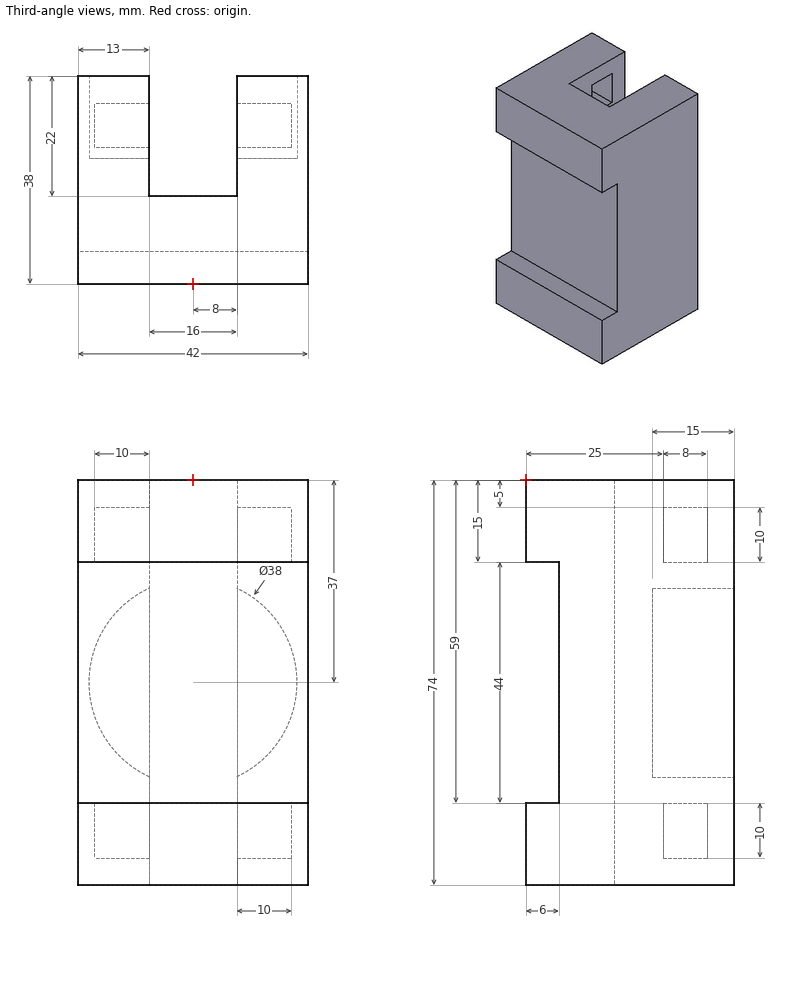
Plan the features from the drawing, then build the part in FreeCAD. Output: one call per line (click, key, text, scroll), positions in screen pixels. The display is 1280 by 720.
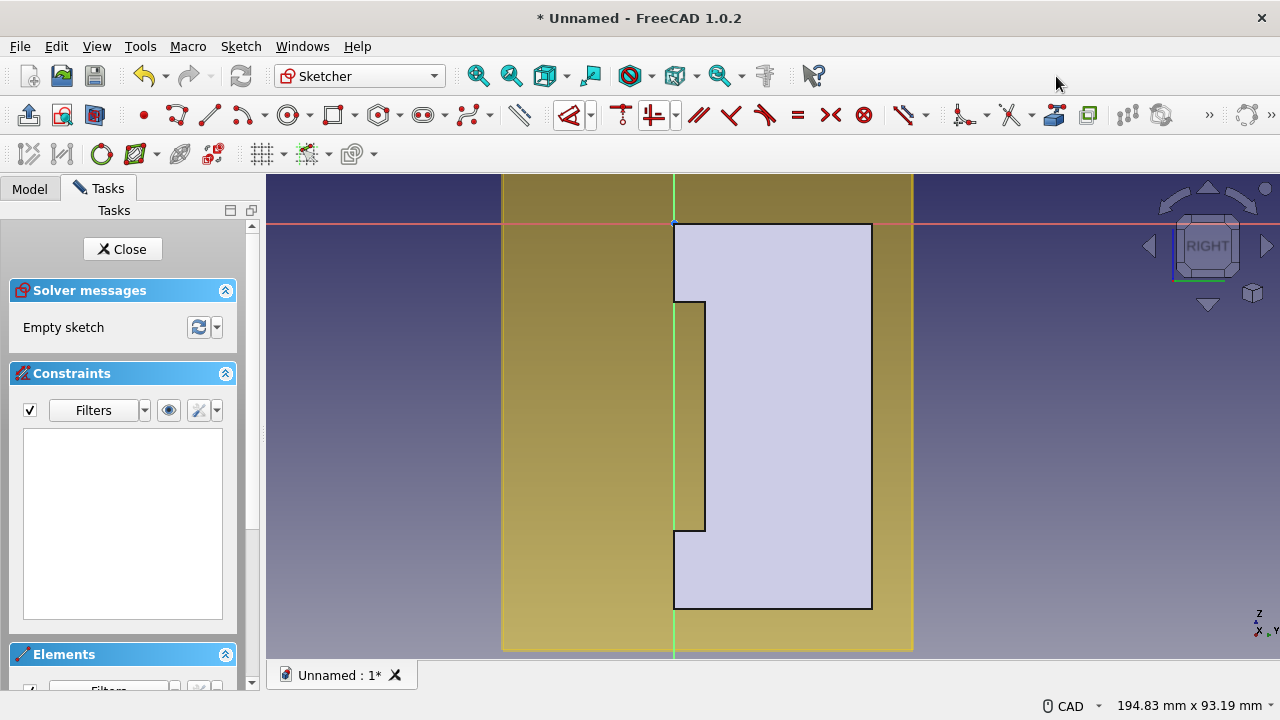
key(q)
key(s)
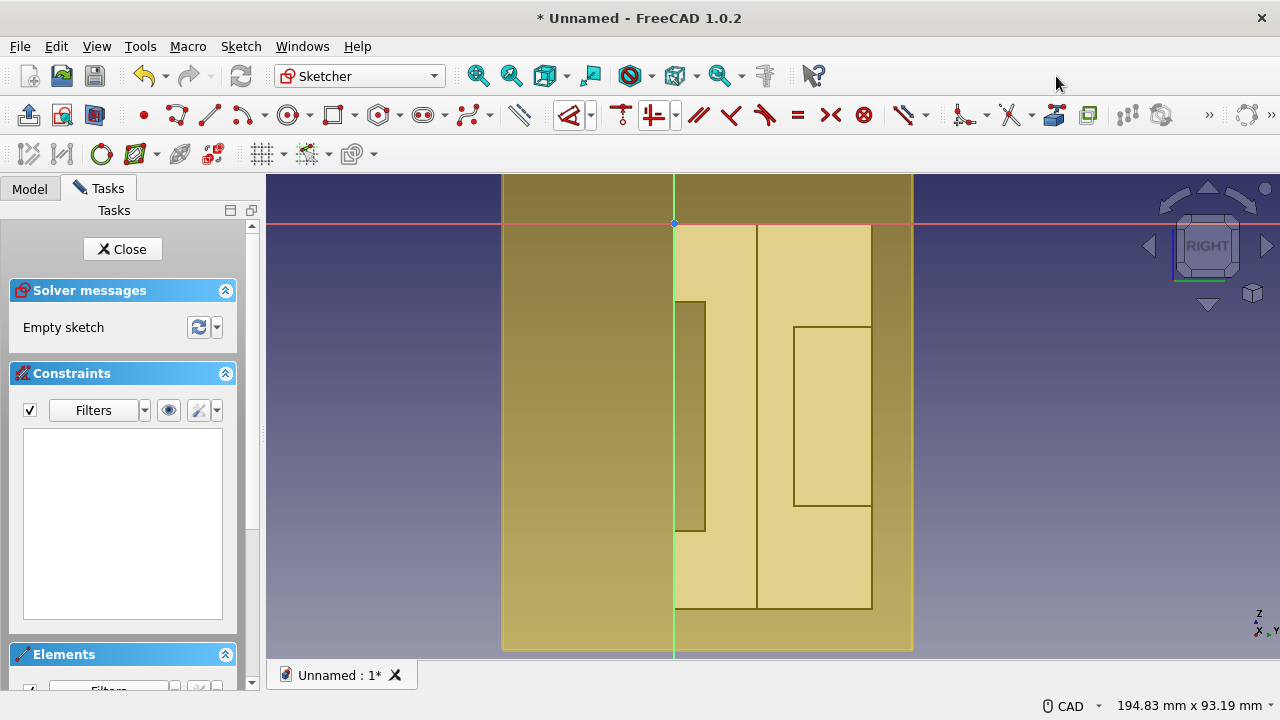
scroll(454, 475, down, 1)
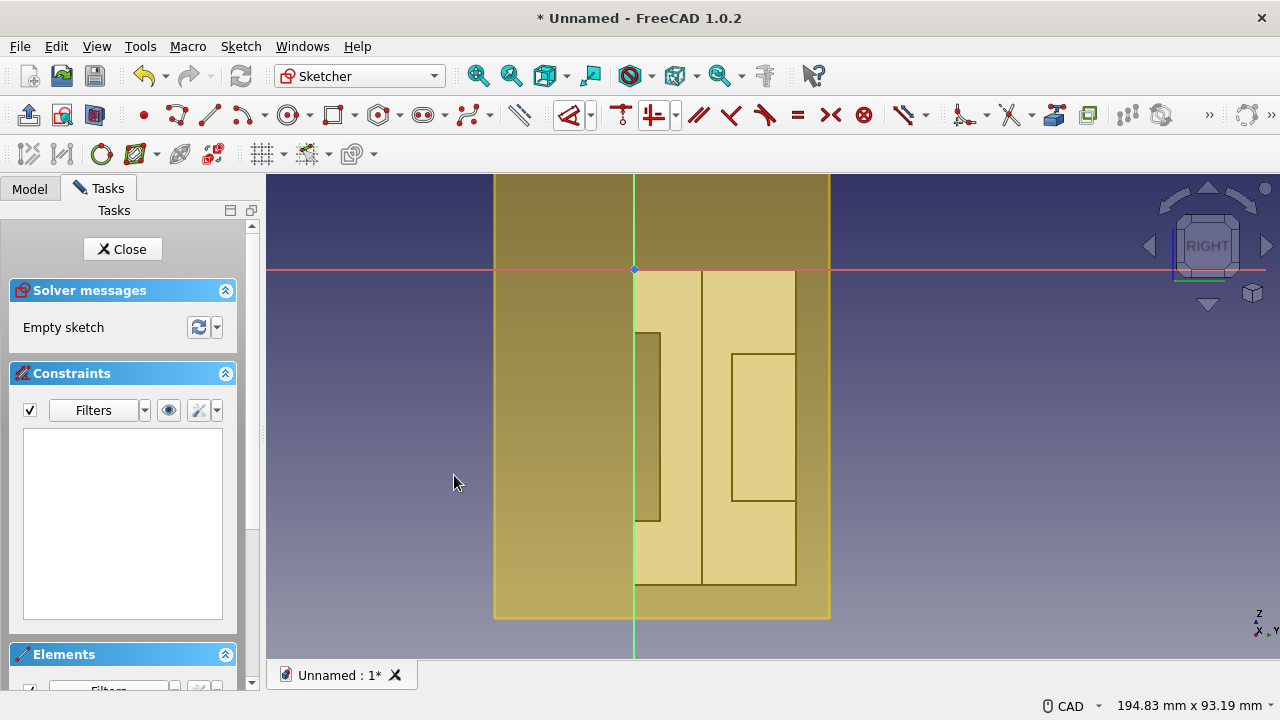
key(g)
key(r)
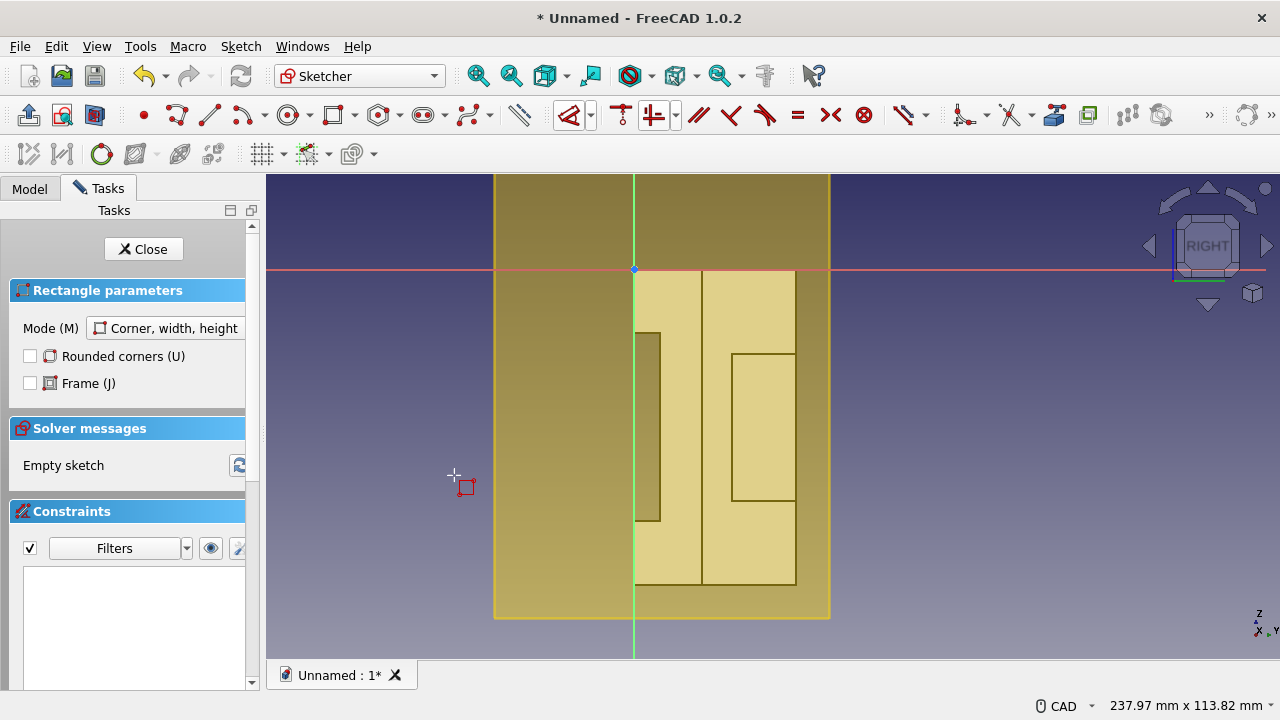
click(741, 291)
move(775, 333)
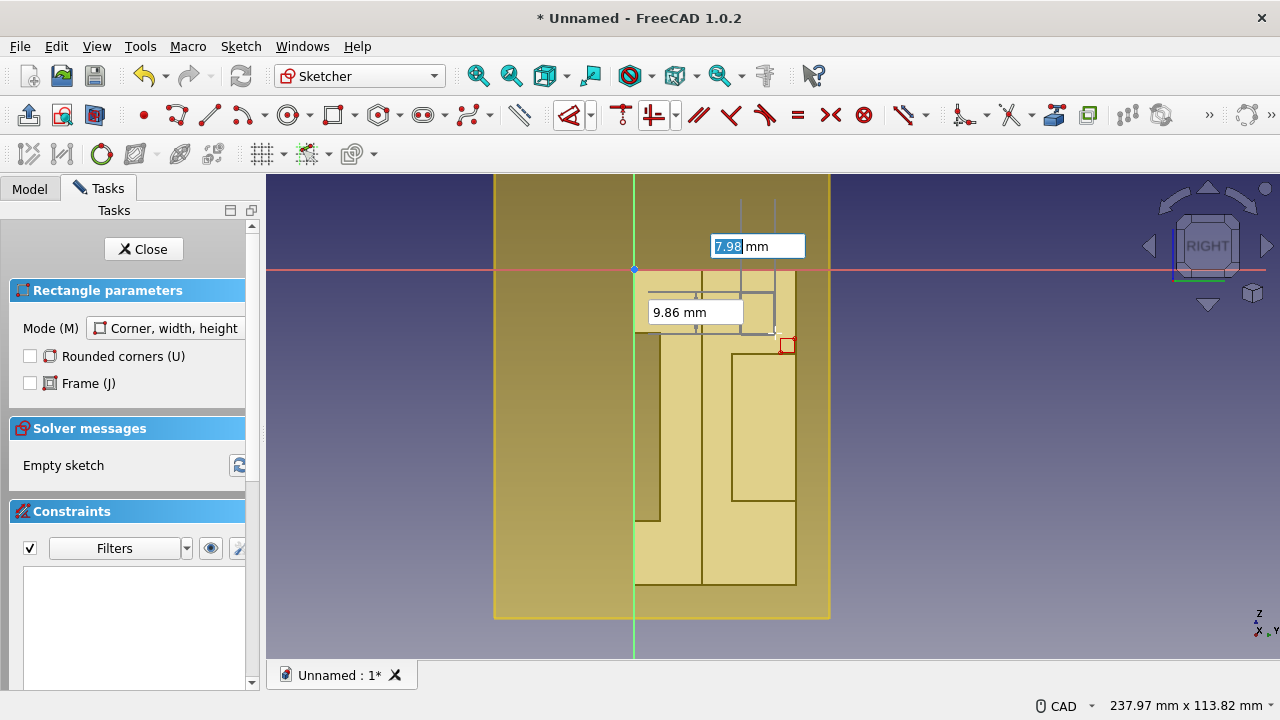
text(8)
key(Tab)
text(10)
key(Return)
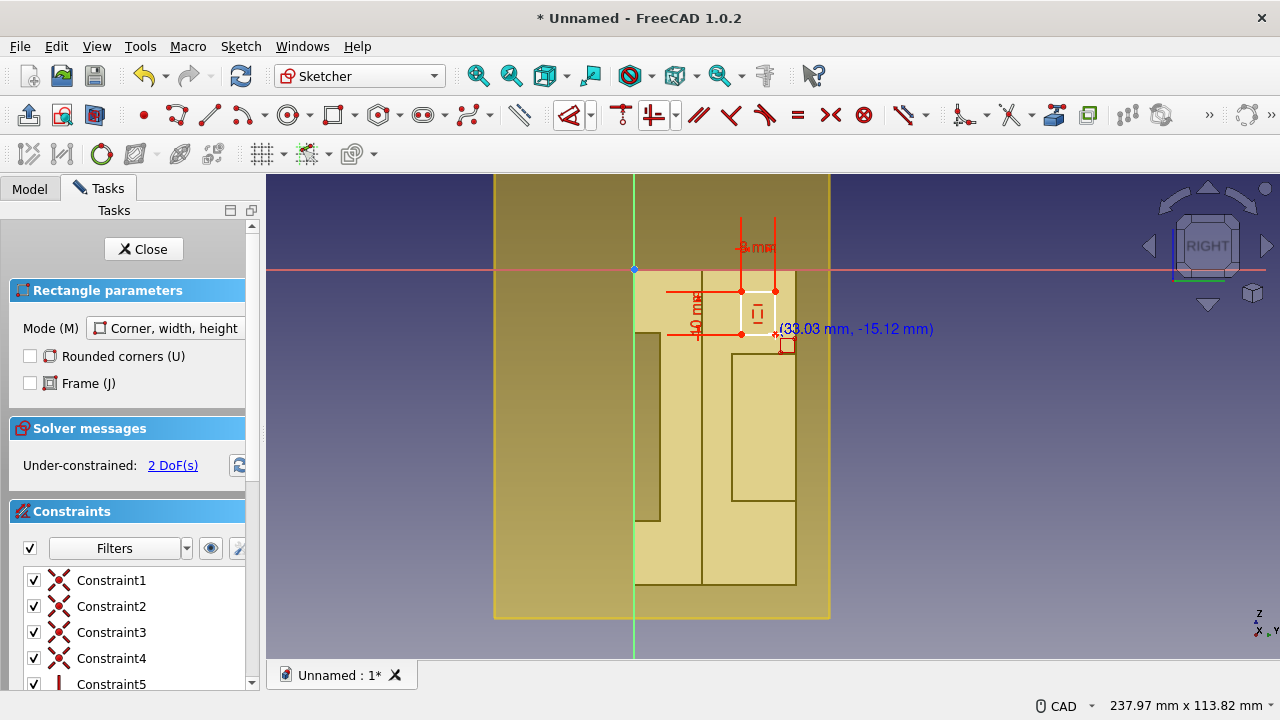
click(741, 521)
move(775, 564)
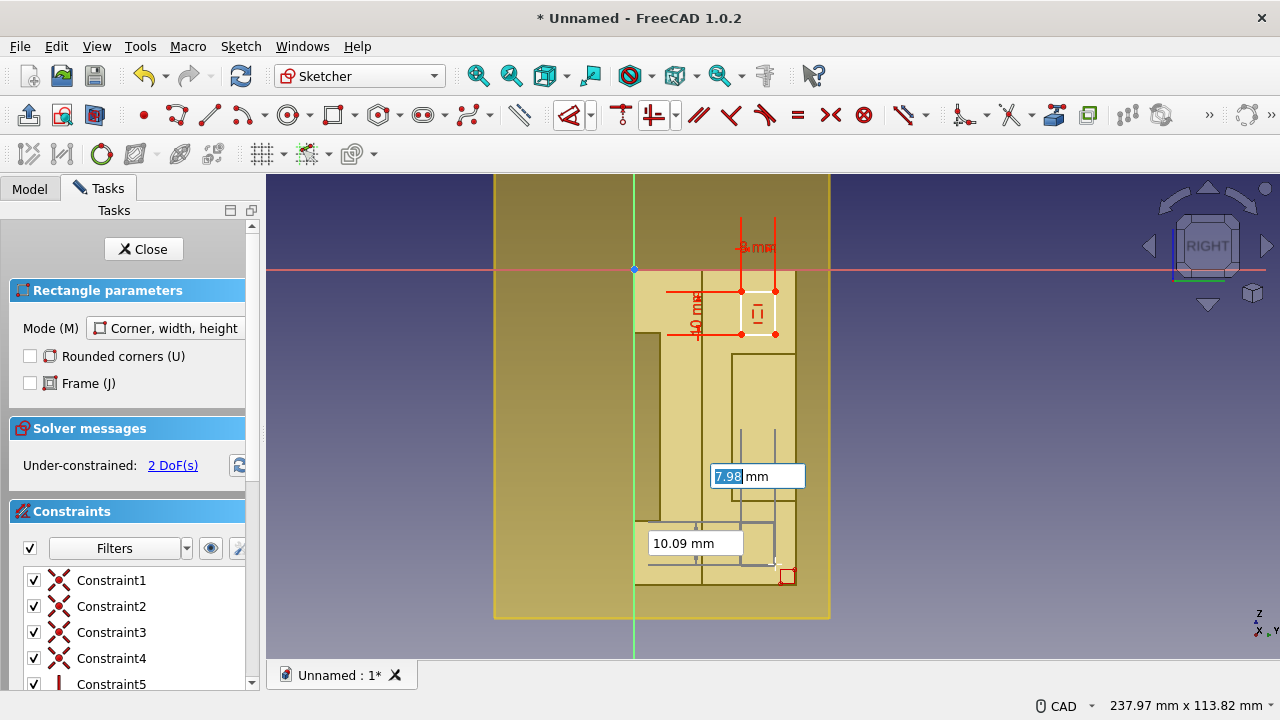
text(8)
key(Tab)
text(10)
key(Return)
key(Escape)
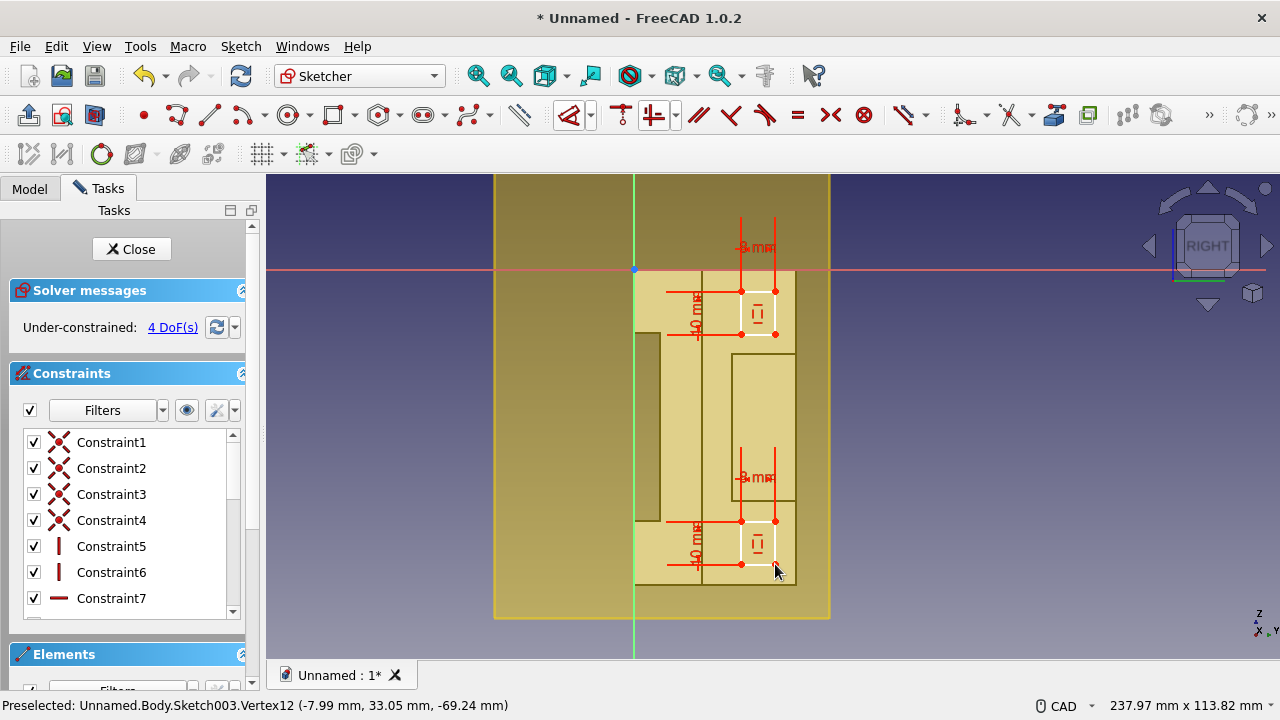
scroll(741, 292, up, 4)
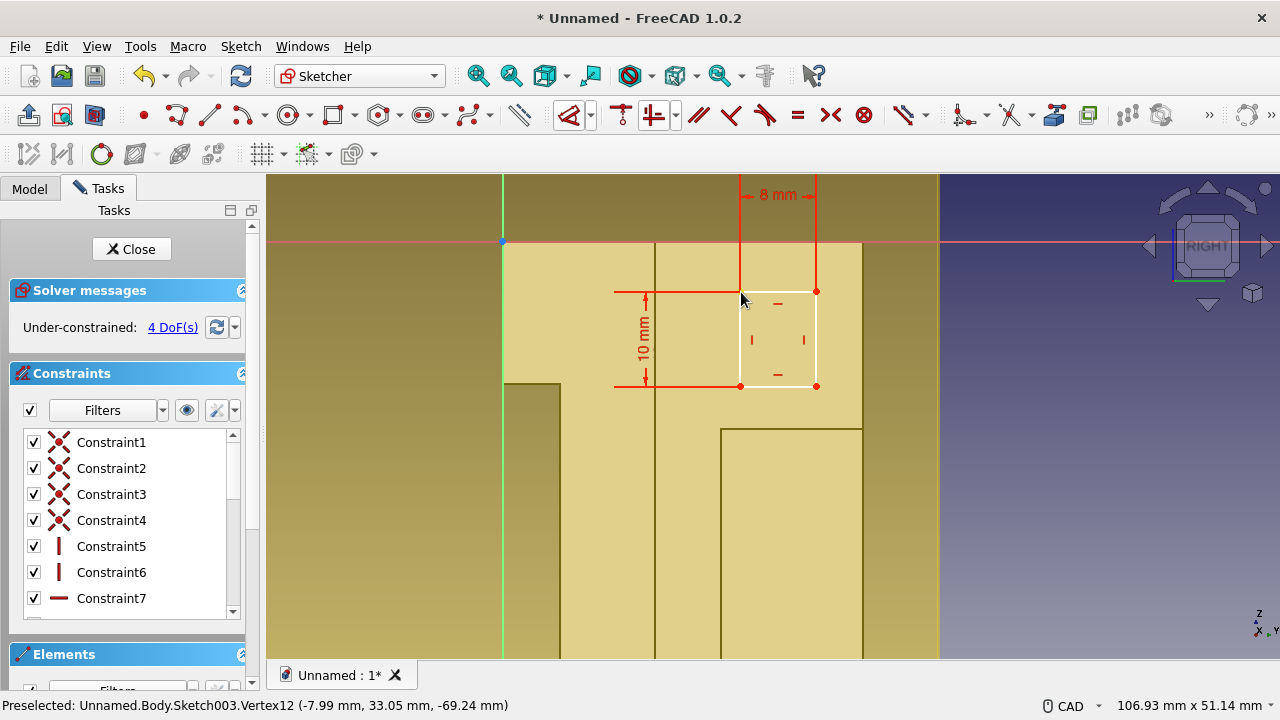
click(740, 292)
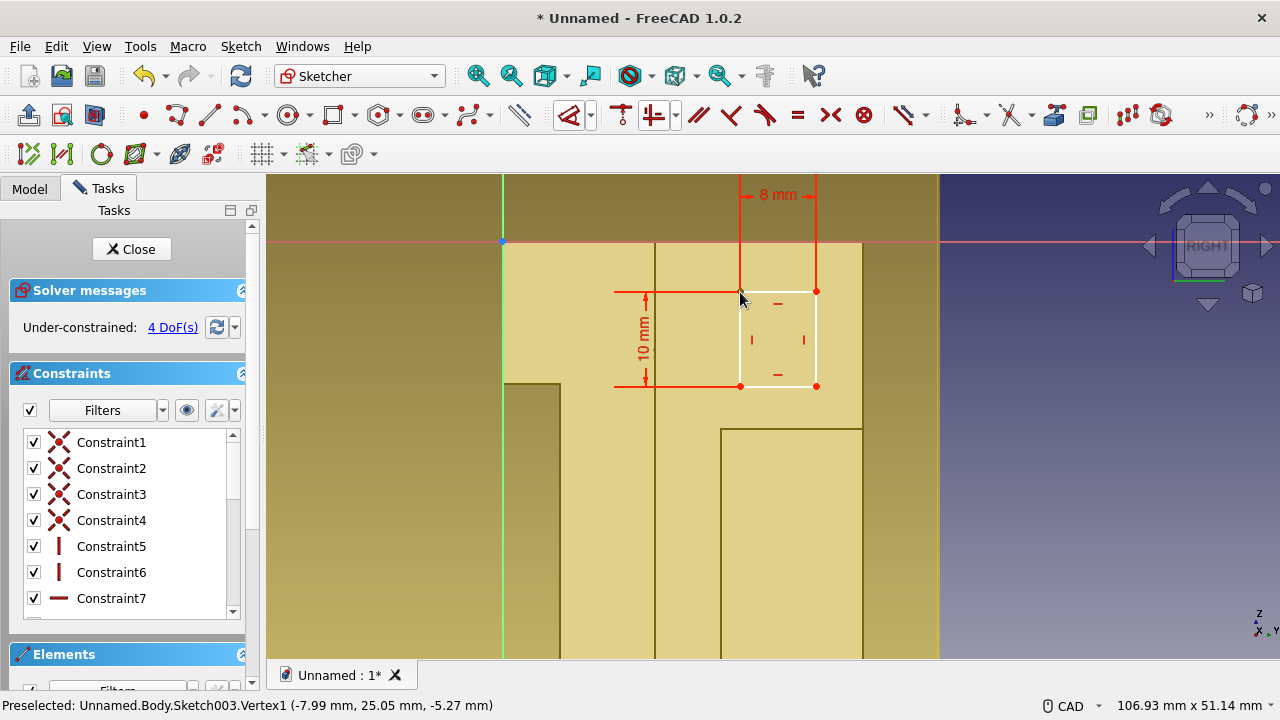
key(i)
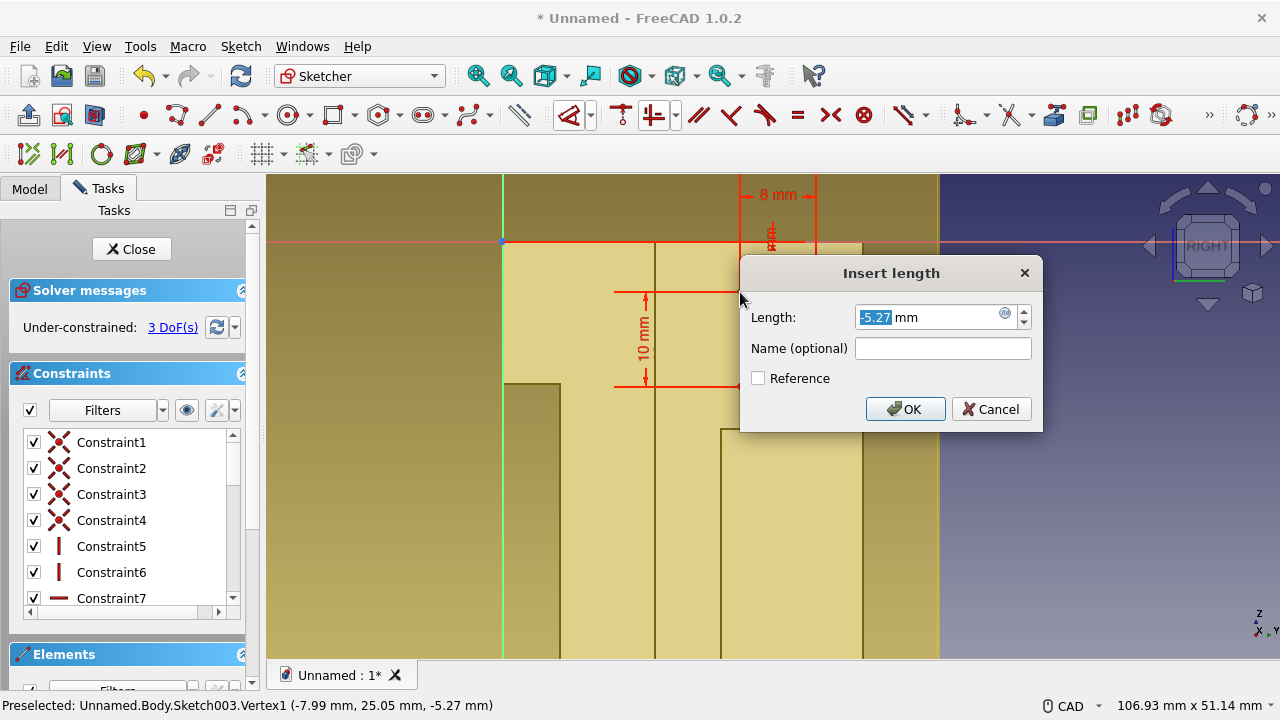
text(-5)
key(Return)